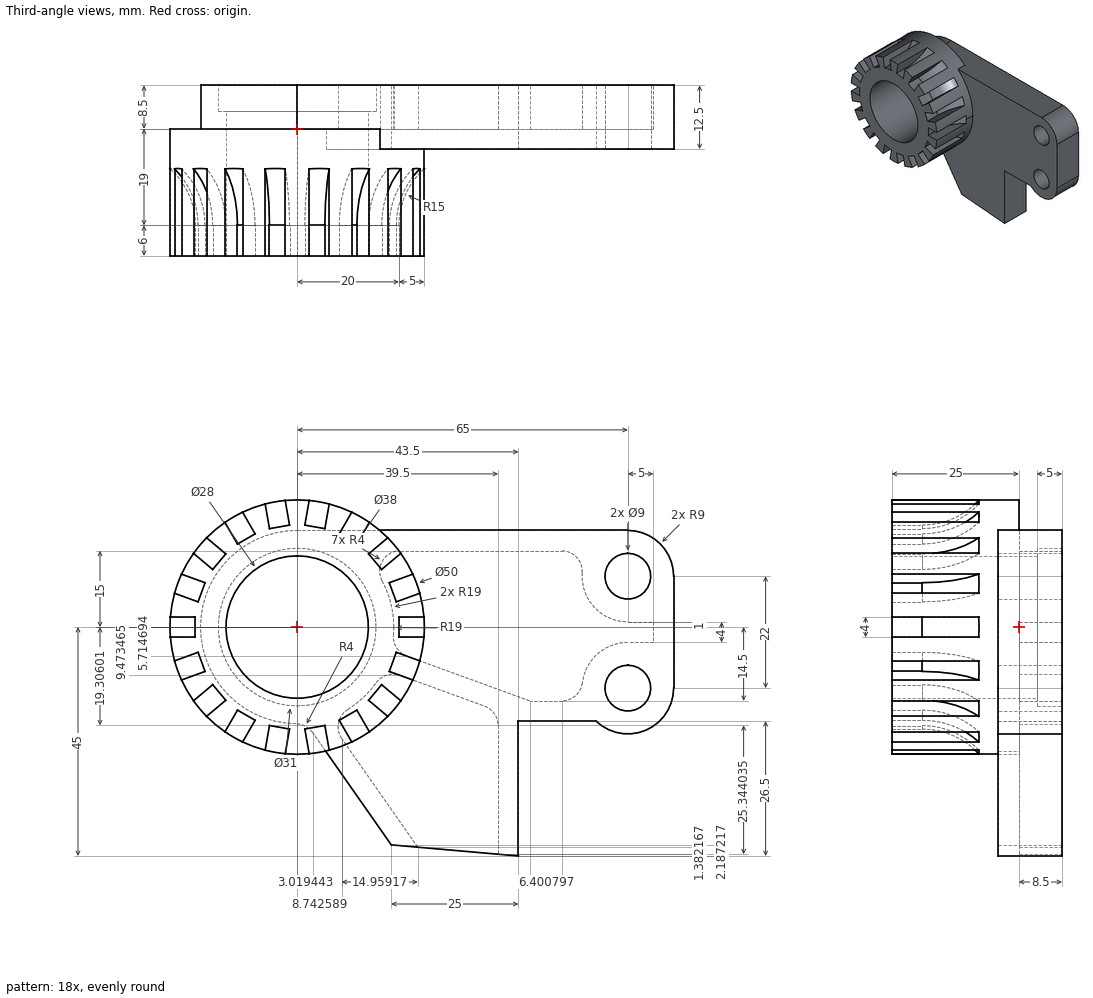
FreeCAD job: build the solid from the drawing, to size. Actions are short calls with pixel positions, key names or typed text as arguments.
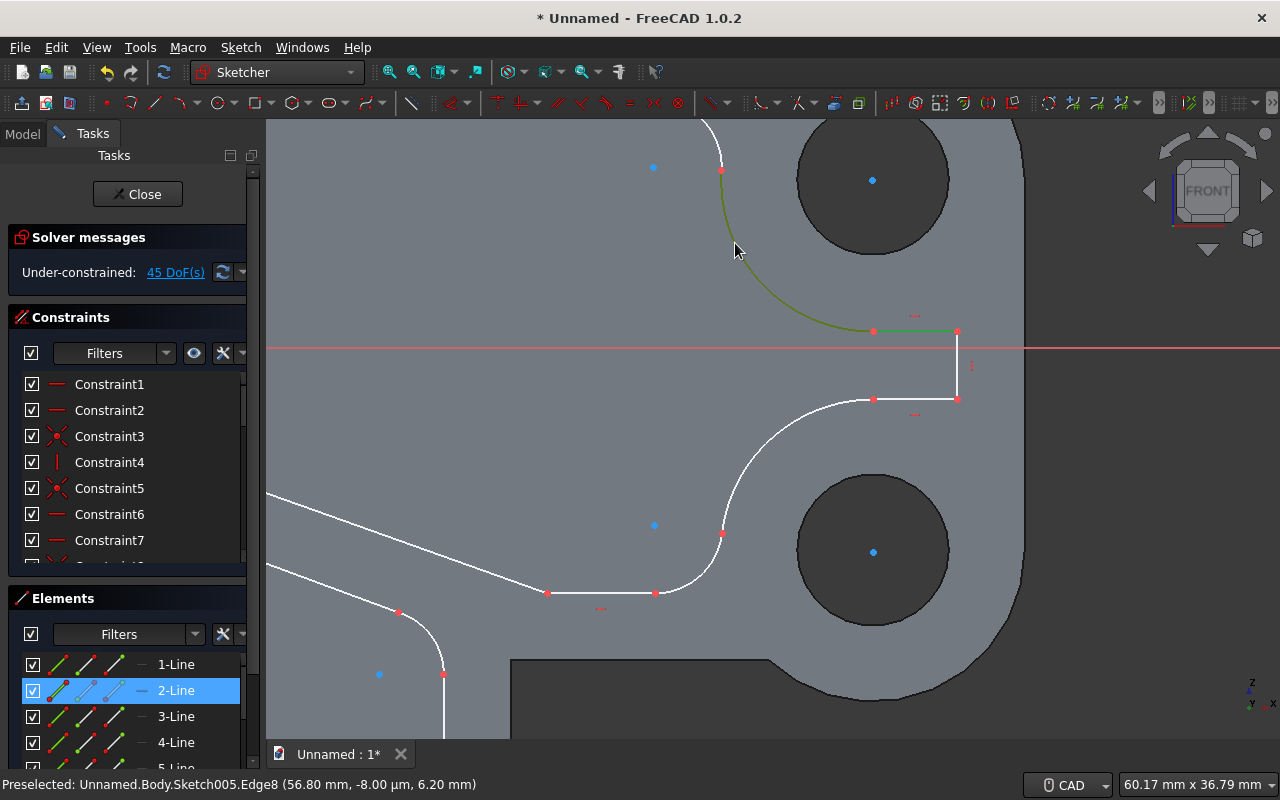
click(606, 104)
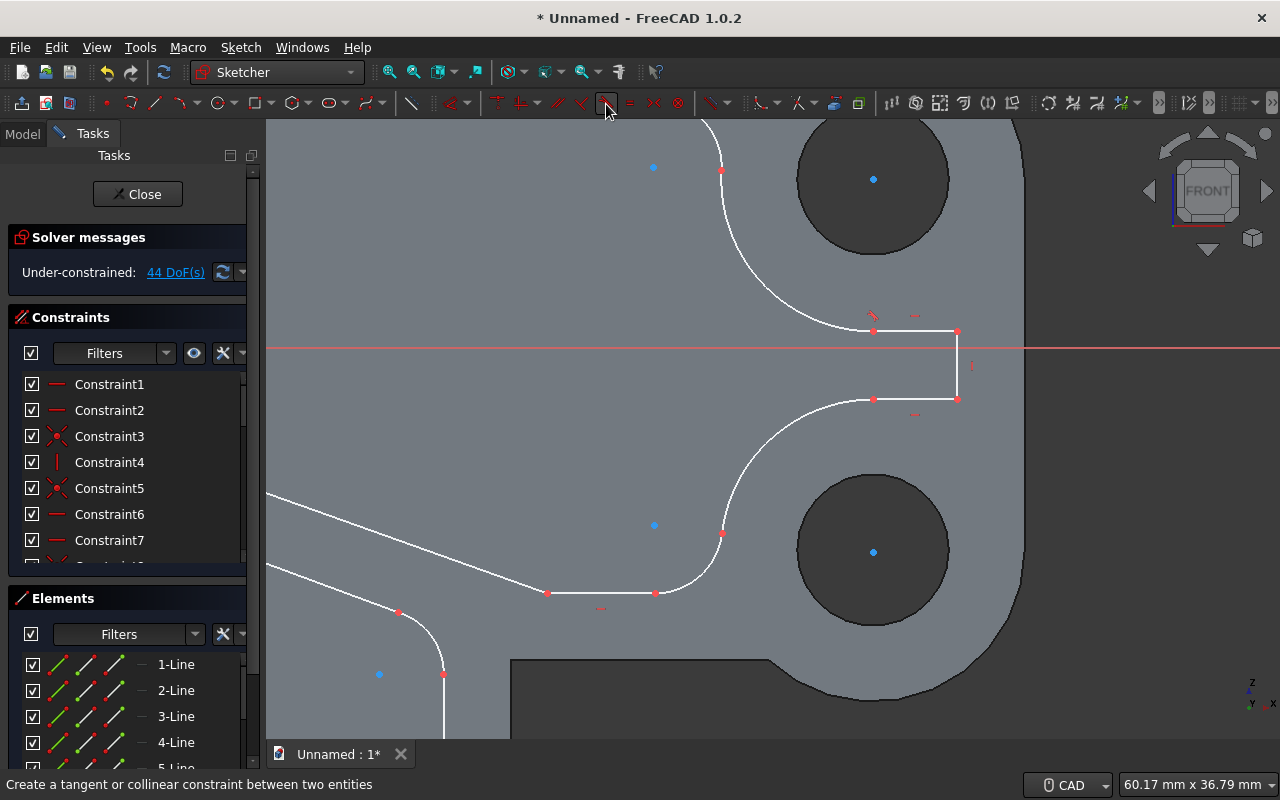
click(932, 399)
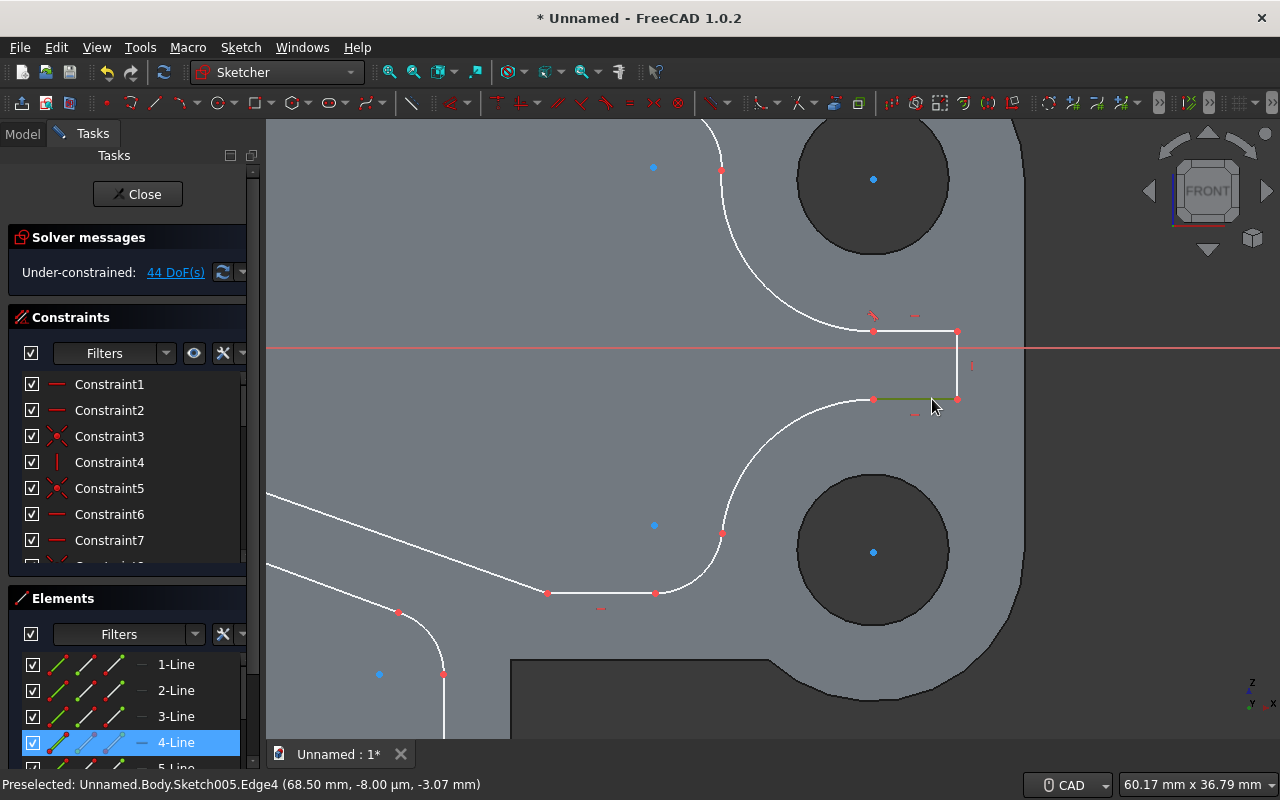
click(809, 414)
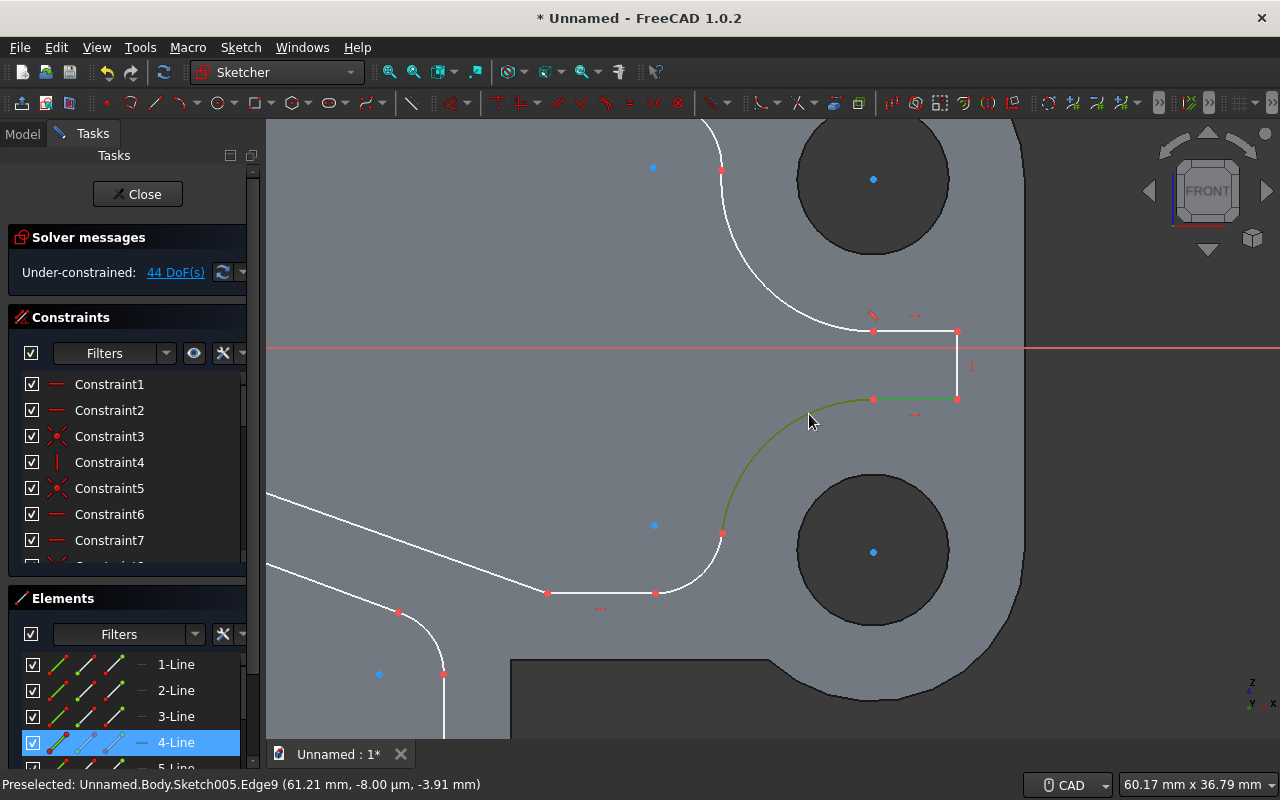
click(606, 104)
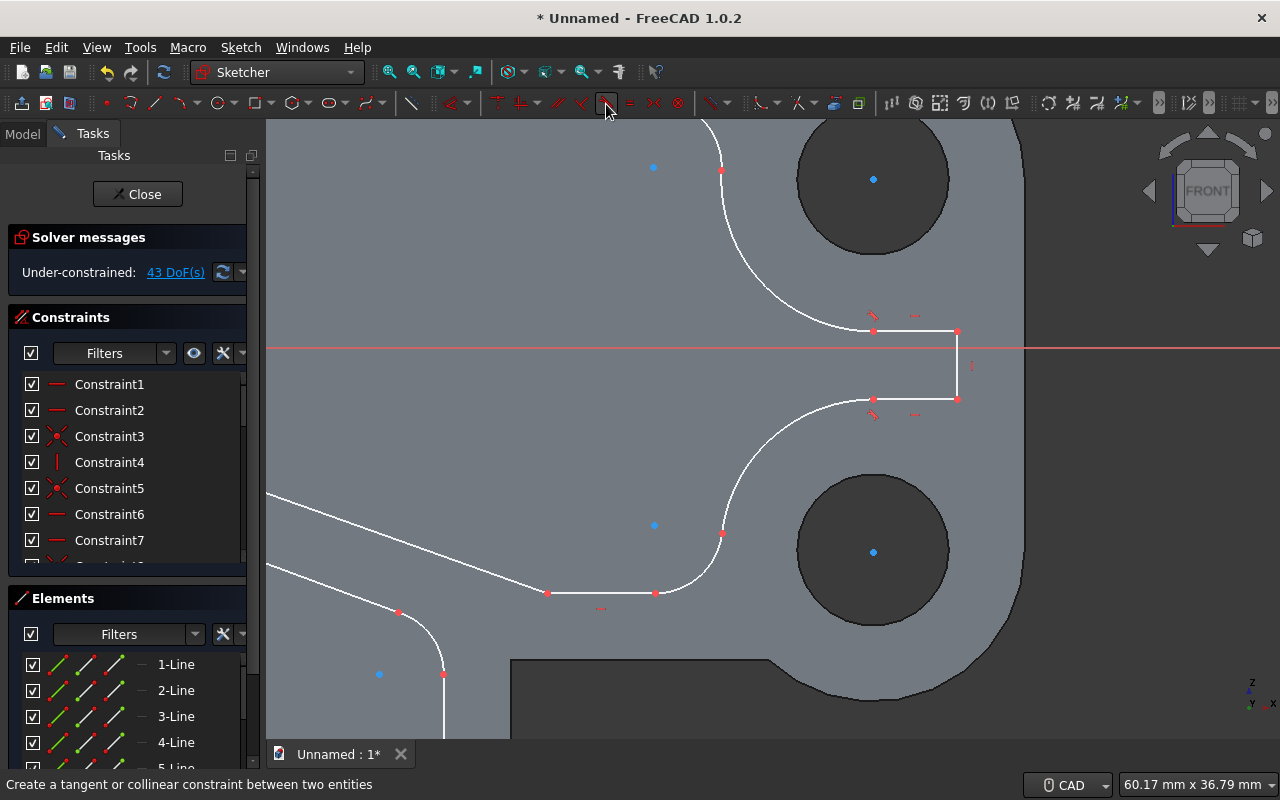
click(623, 593)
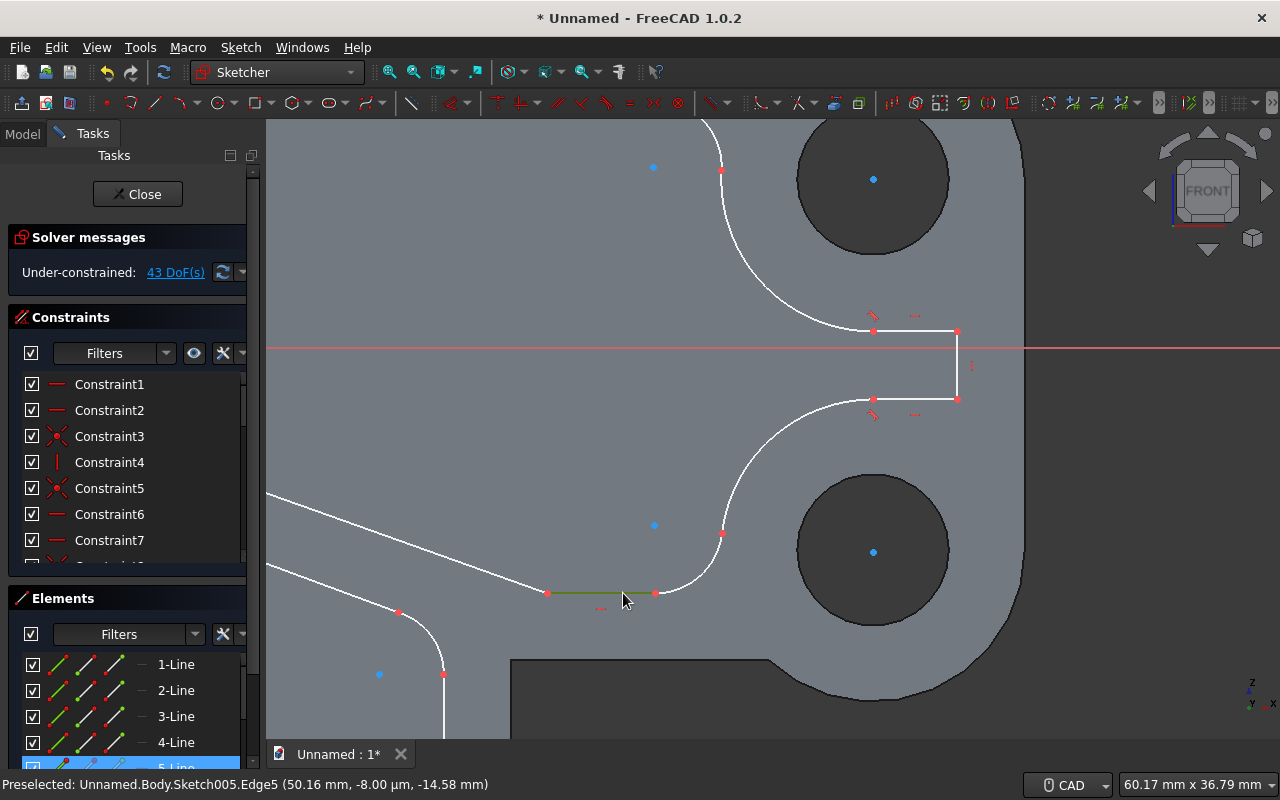
click(684, 587)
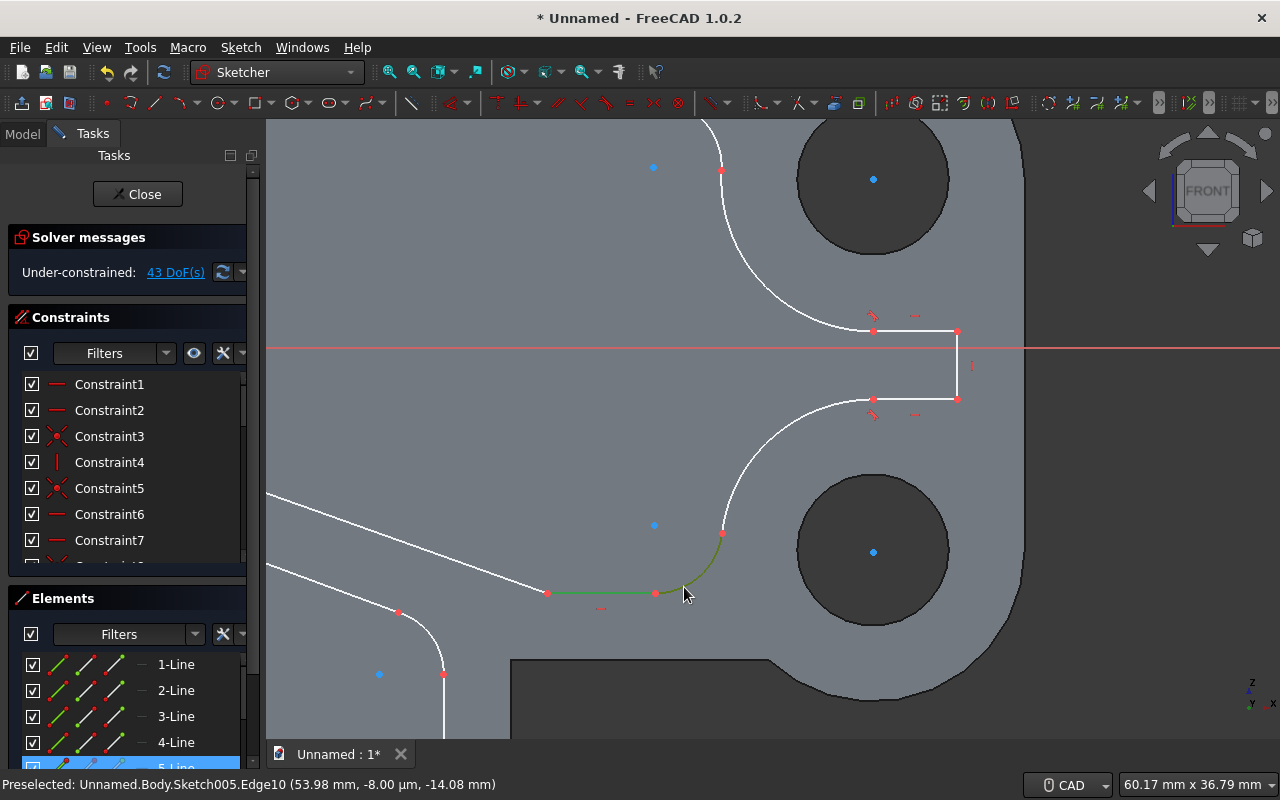
click(606, 104)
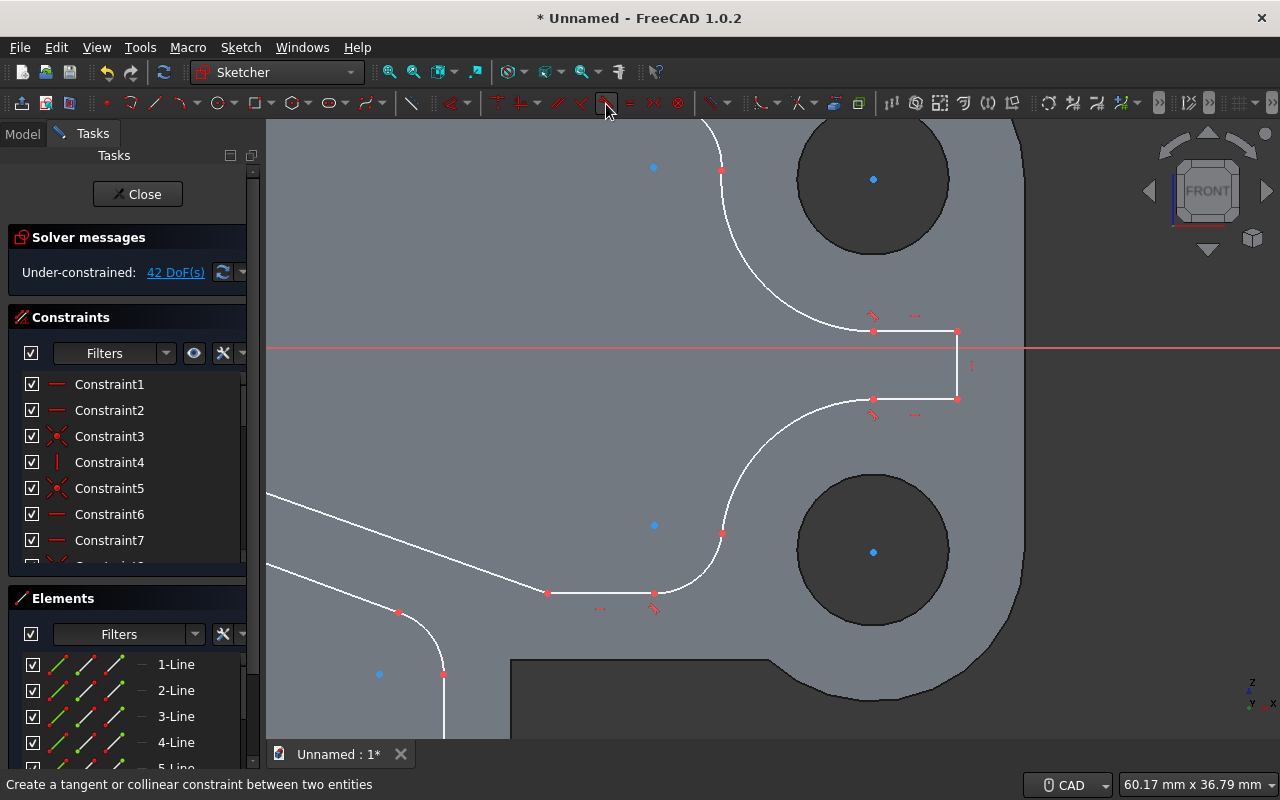
click(425, 550)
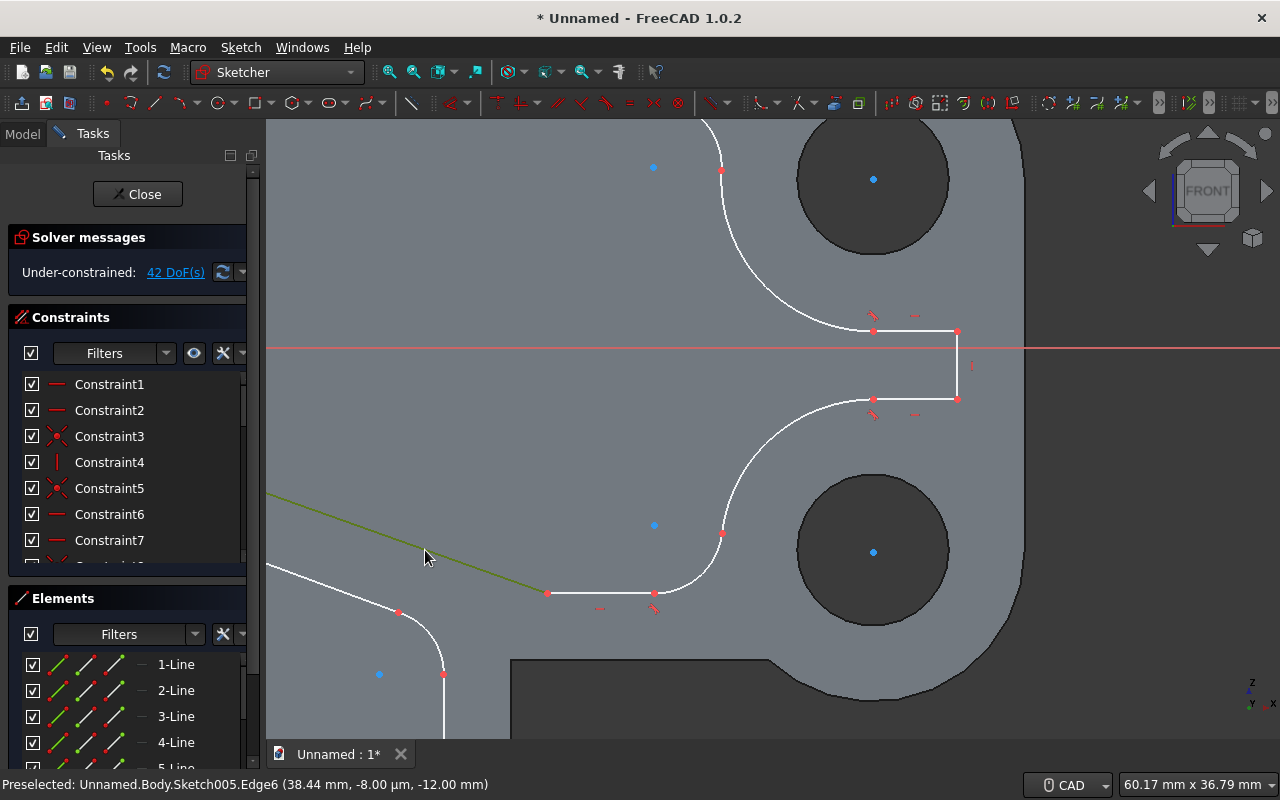
scroll(901, 331, down, 5)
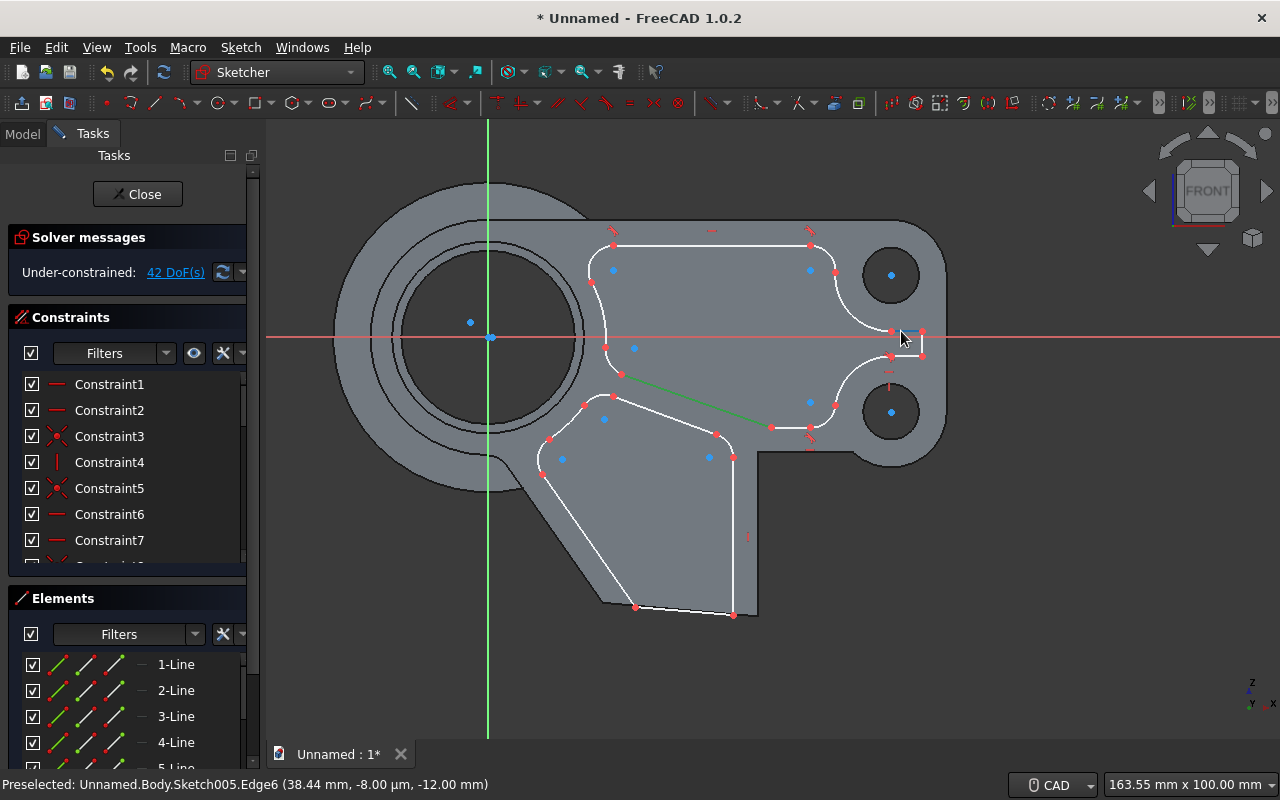
scroll(607, 357, up, 2)